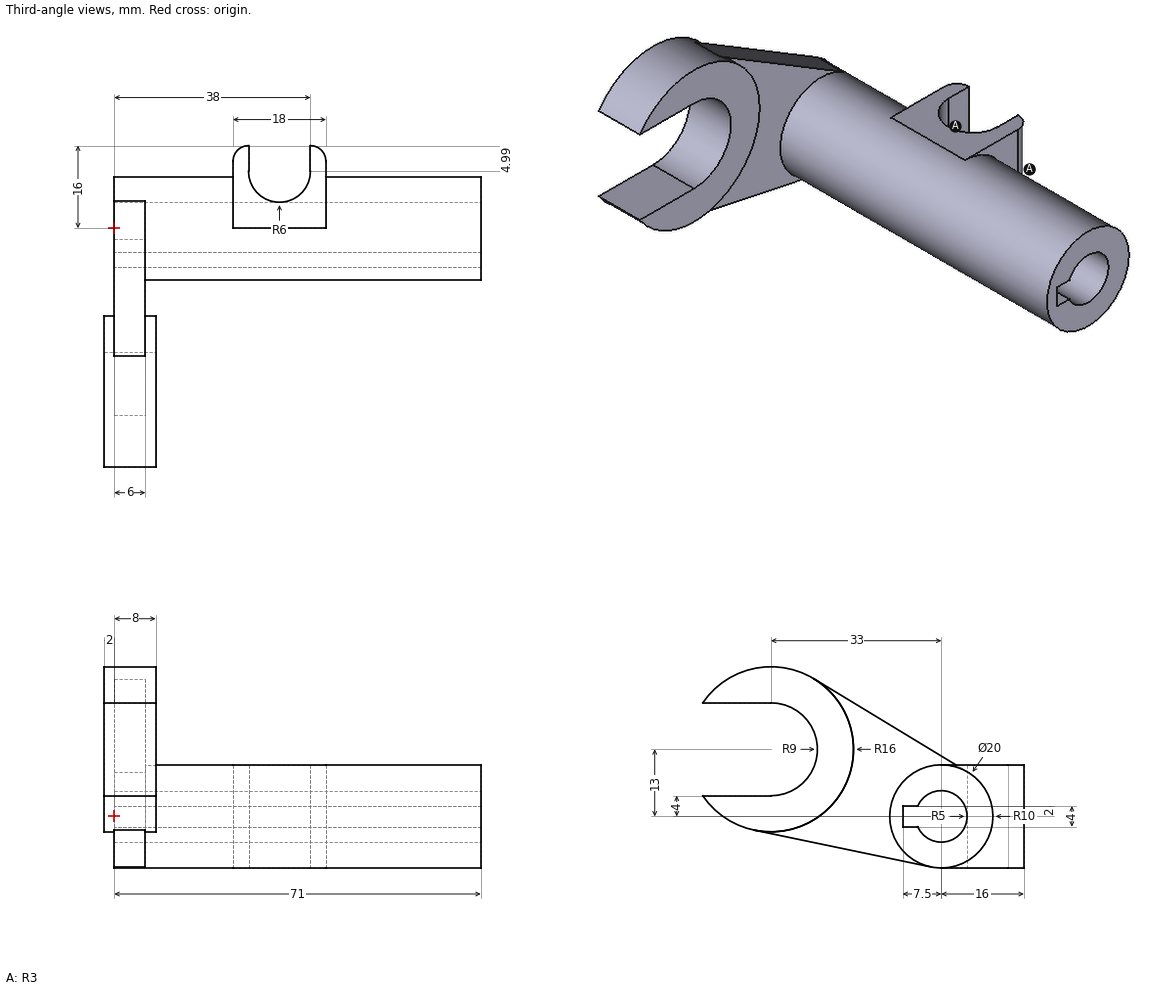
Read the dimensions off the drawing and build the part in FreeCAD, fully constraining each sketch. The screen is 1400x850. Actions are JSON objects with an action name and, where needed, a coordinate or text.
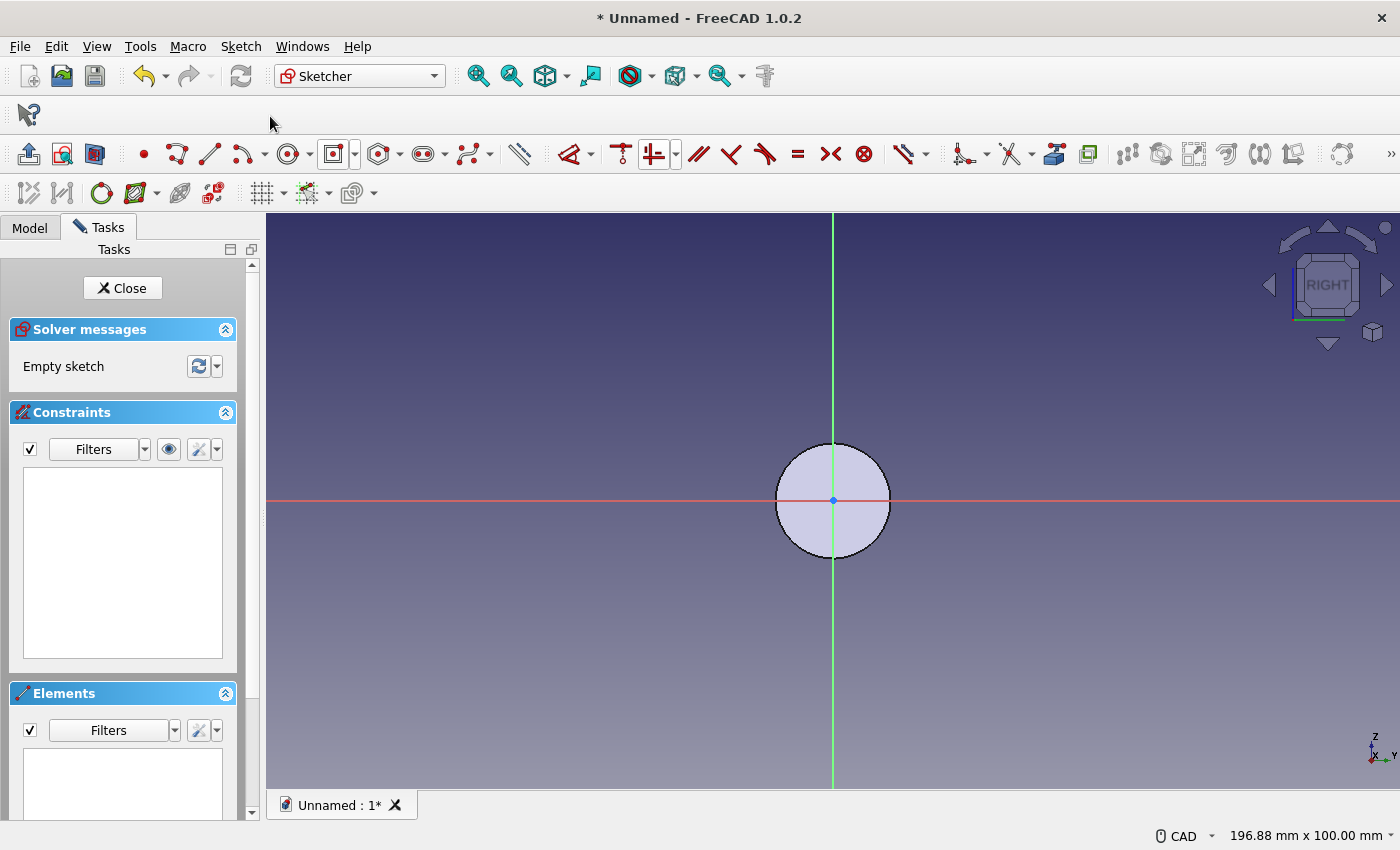
{"action": "scroll", "coordinate": [833, 501], "scroll_direction": "up", "scroll_amount": 11}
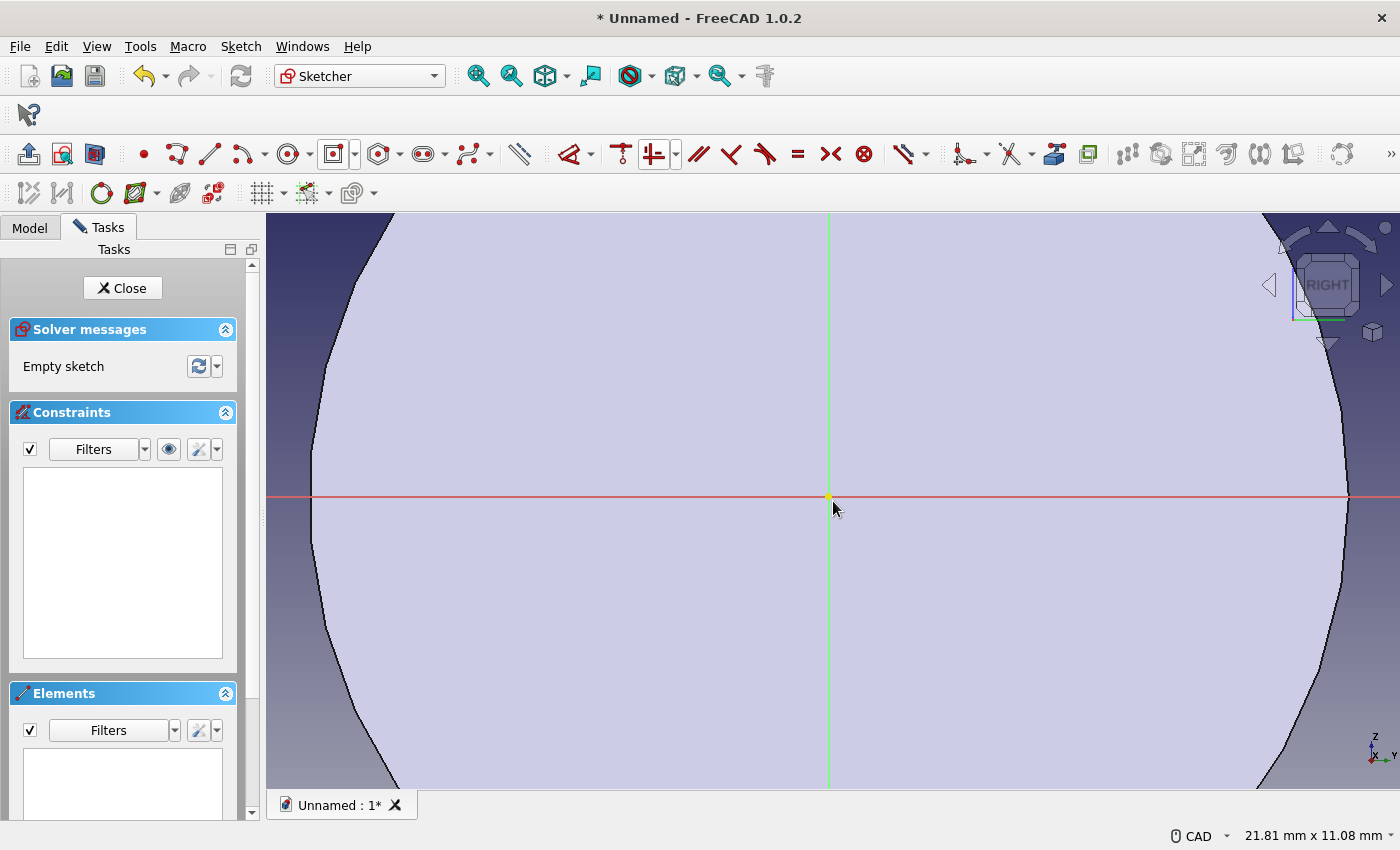
{"action": "key", "text": "g m"}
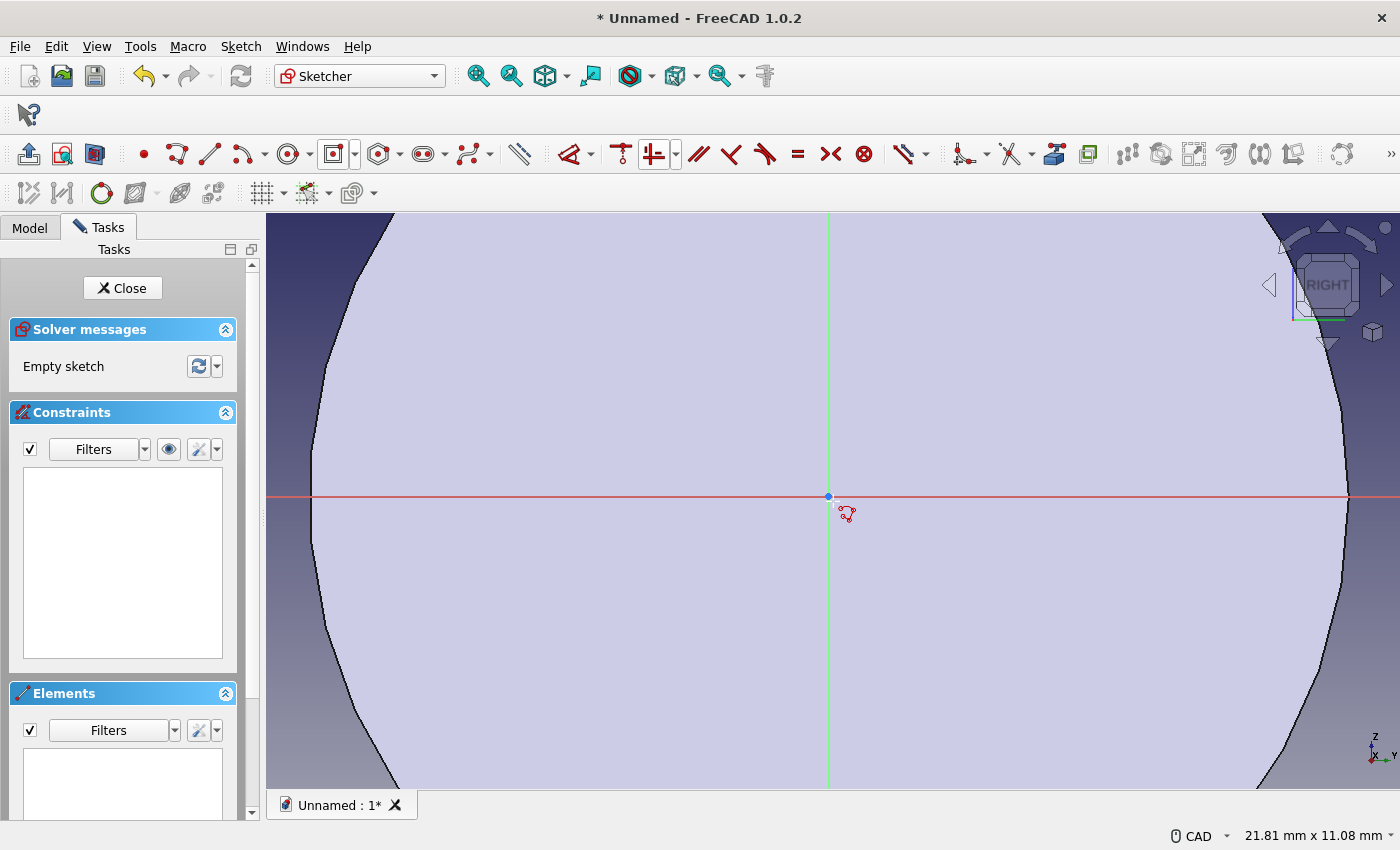
{"action": "left_click", "coordinate": [591, 393]}
{"action": "left_click", "coordinate": [439, 393]}
{"action": "left_click", "coordinate": [439, 601]}
{"action": "left_click", "coordinate": [591, 601]}
{"action": "right_click", "coordinate": [591, 601]}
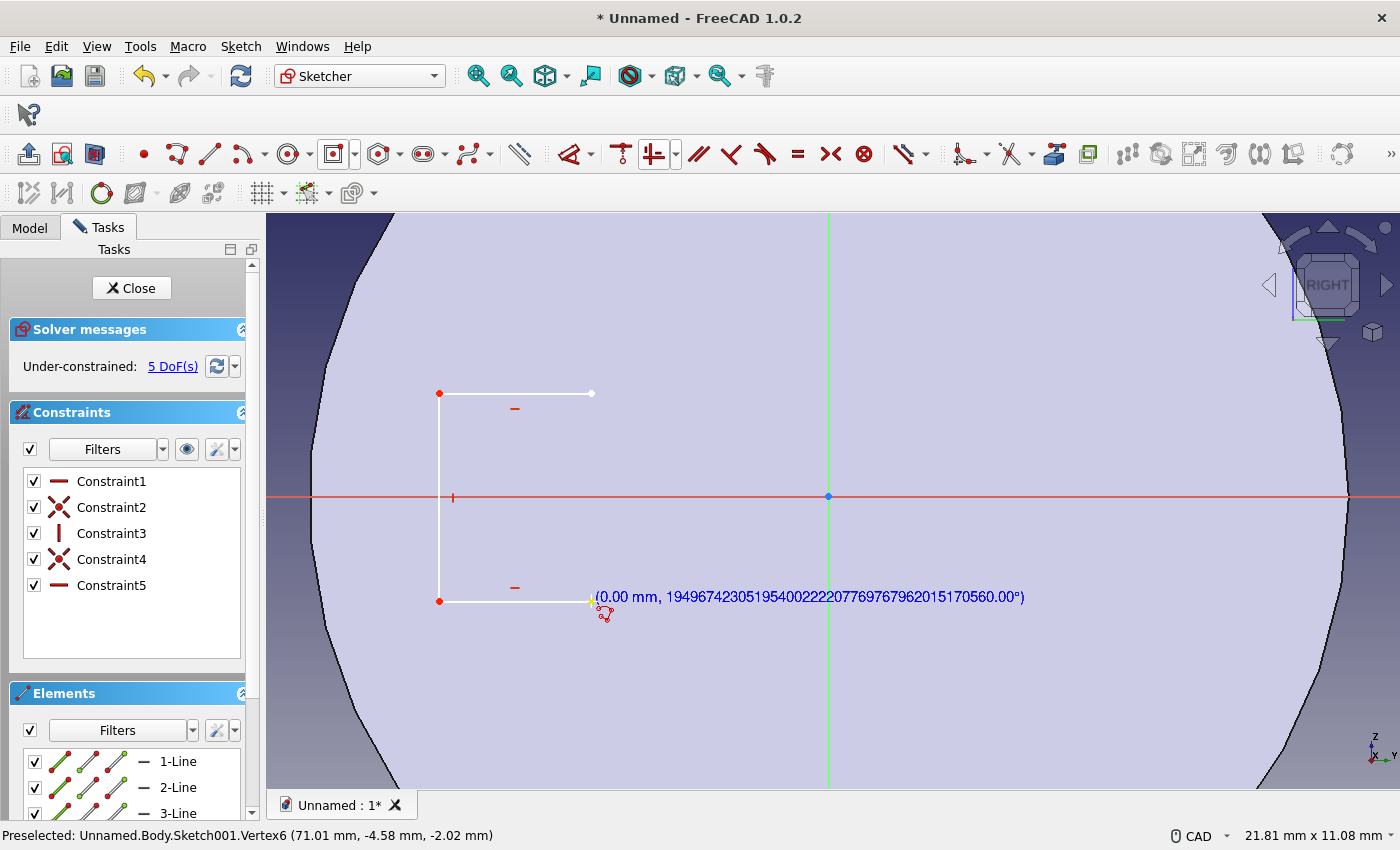
{"action": "key", "text": "g 3 a"}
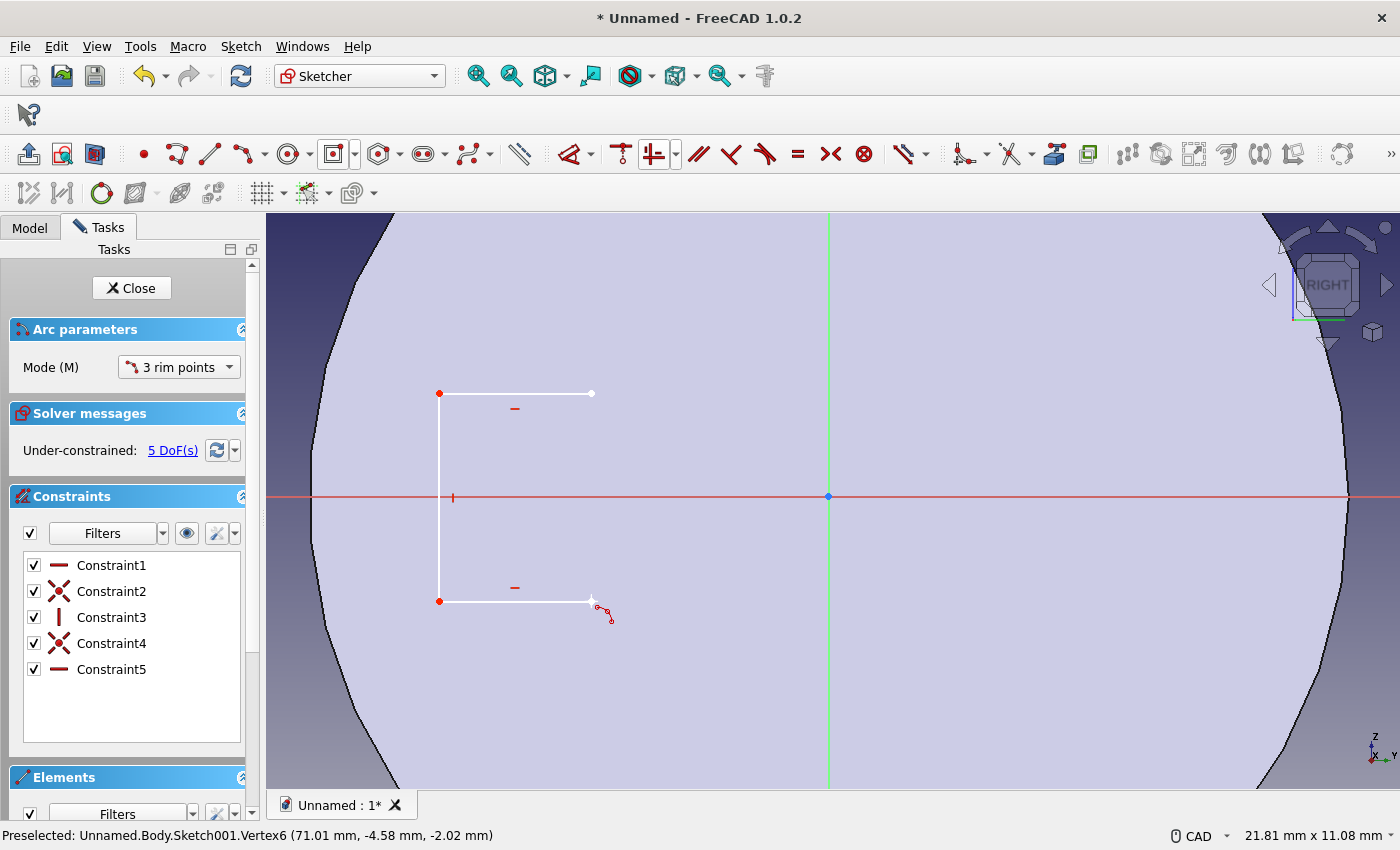
{"action": "left_click", "coordinate": [591, 602]}
{"action": "left_click", "coordinate": [591, 394]}
{"action": "left_click", "coordinate": [1051, 632]}
{"action": "key", "text": "Escape"}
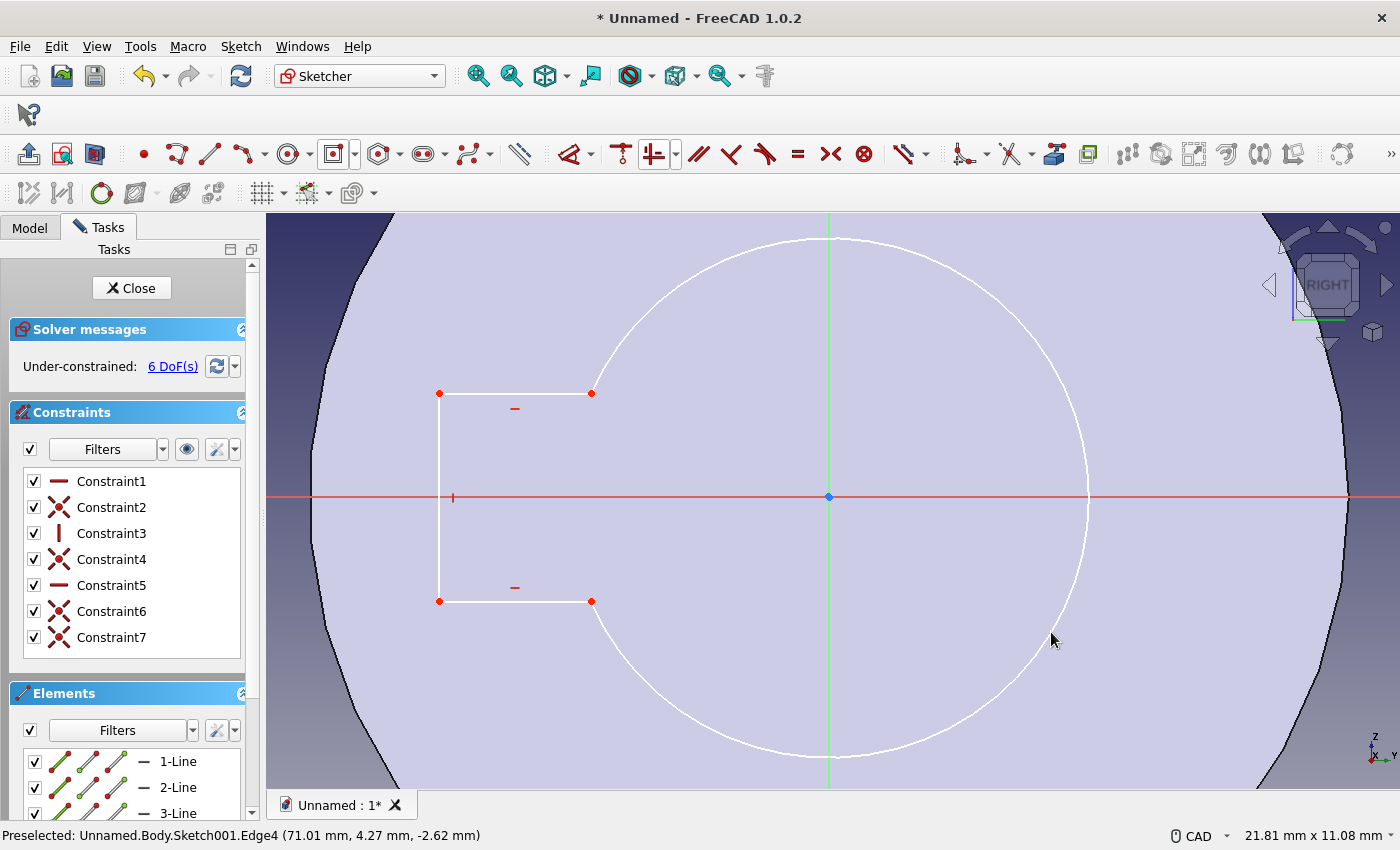
{"action": "left_click_drag", "start_coordinate": [819, 487], "coordinate": [839, 508]}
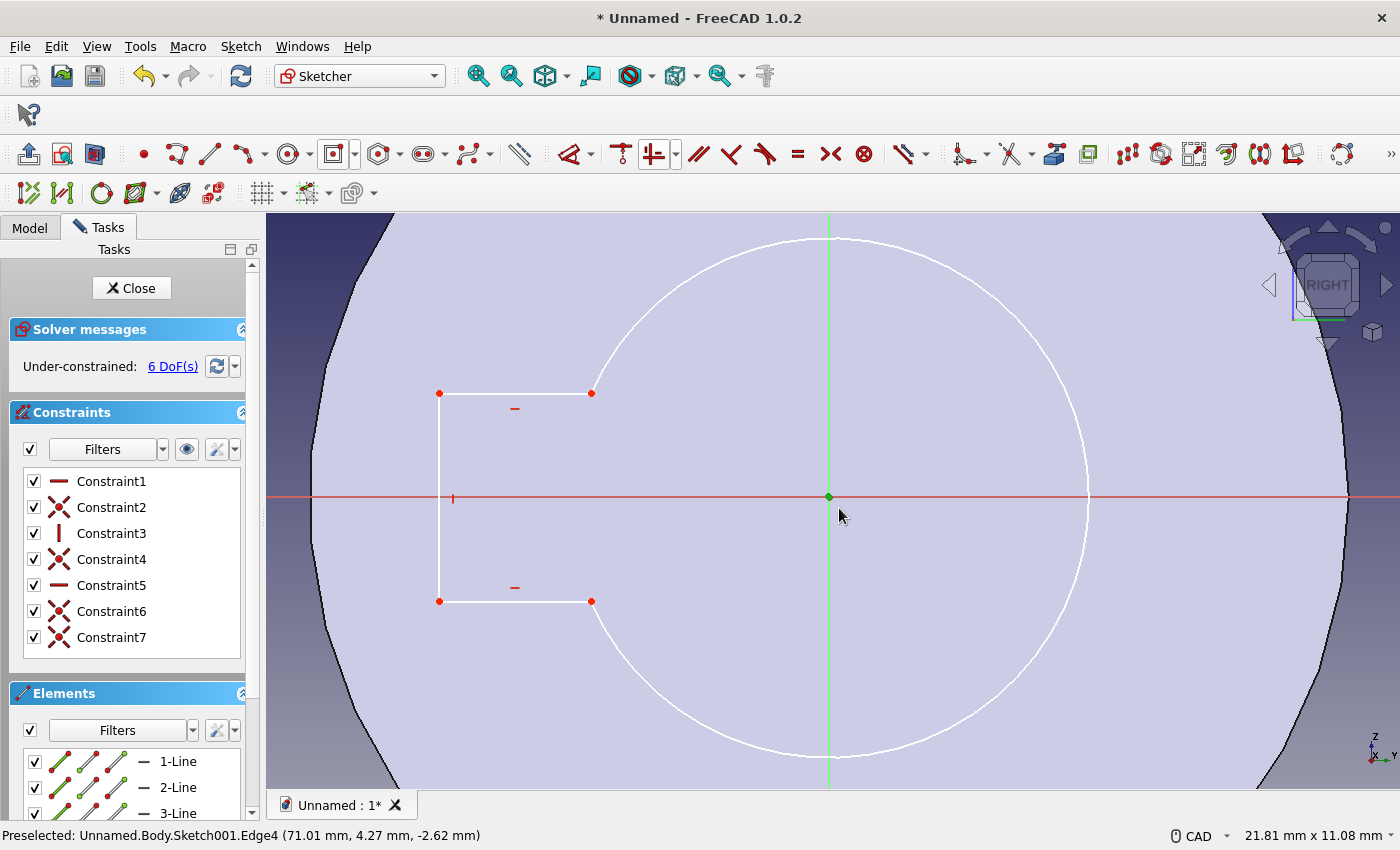
{"action": "key", "text": "c"}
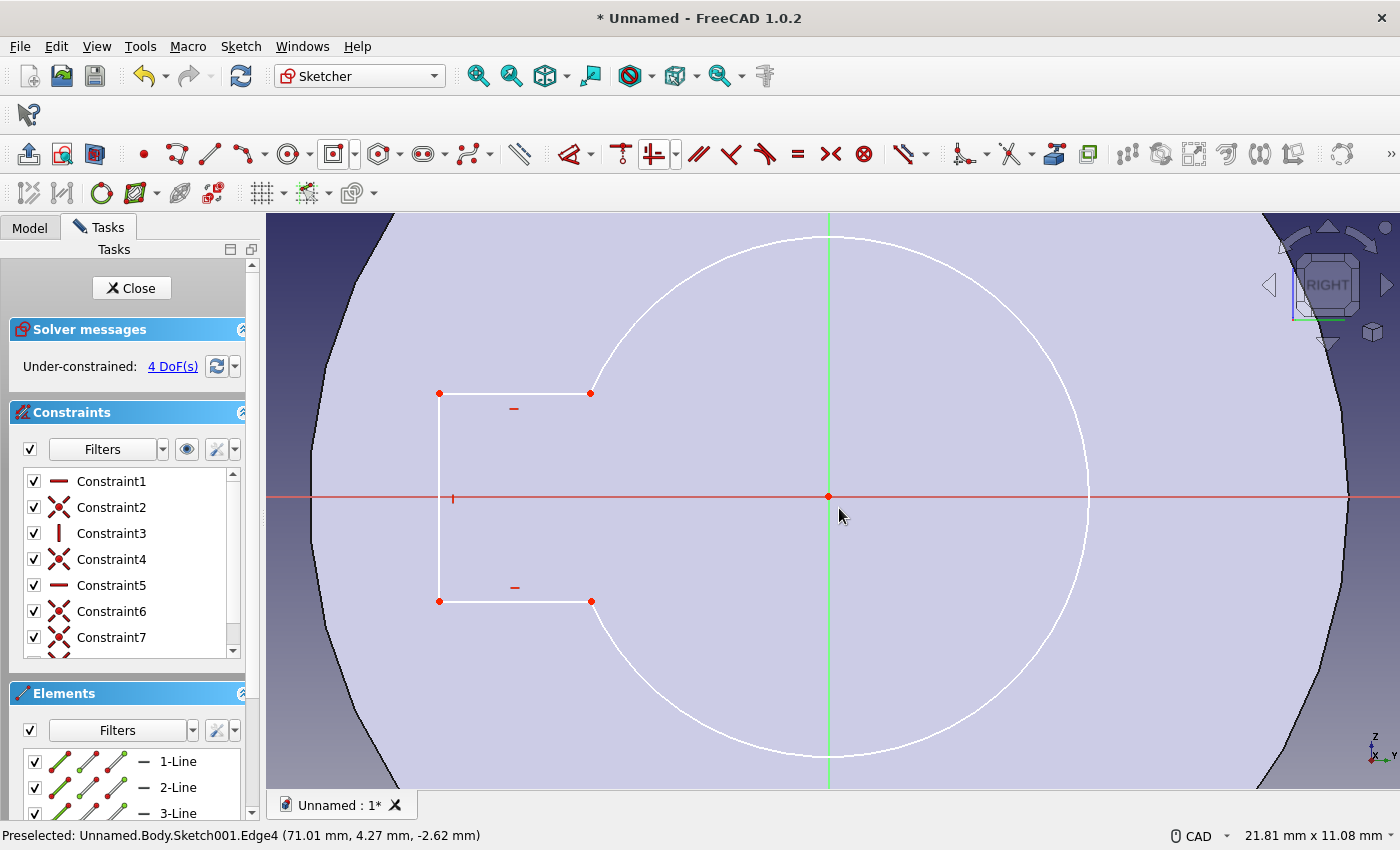
{"action": "key", "text": "d"}